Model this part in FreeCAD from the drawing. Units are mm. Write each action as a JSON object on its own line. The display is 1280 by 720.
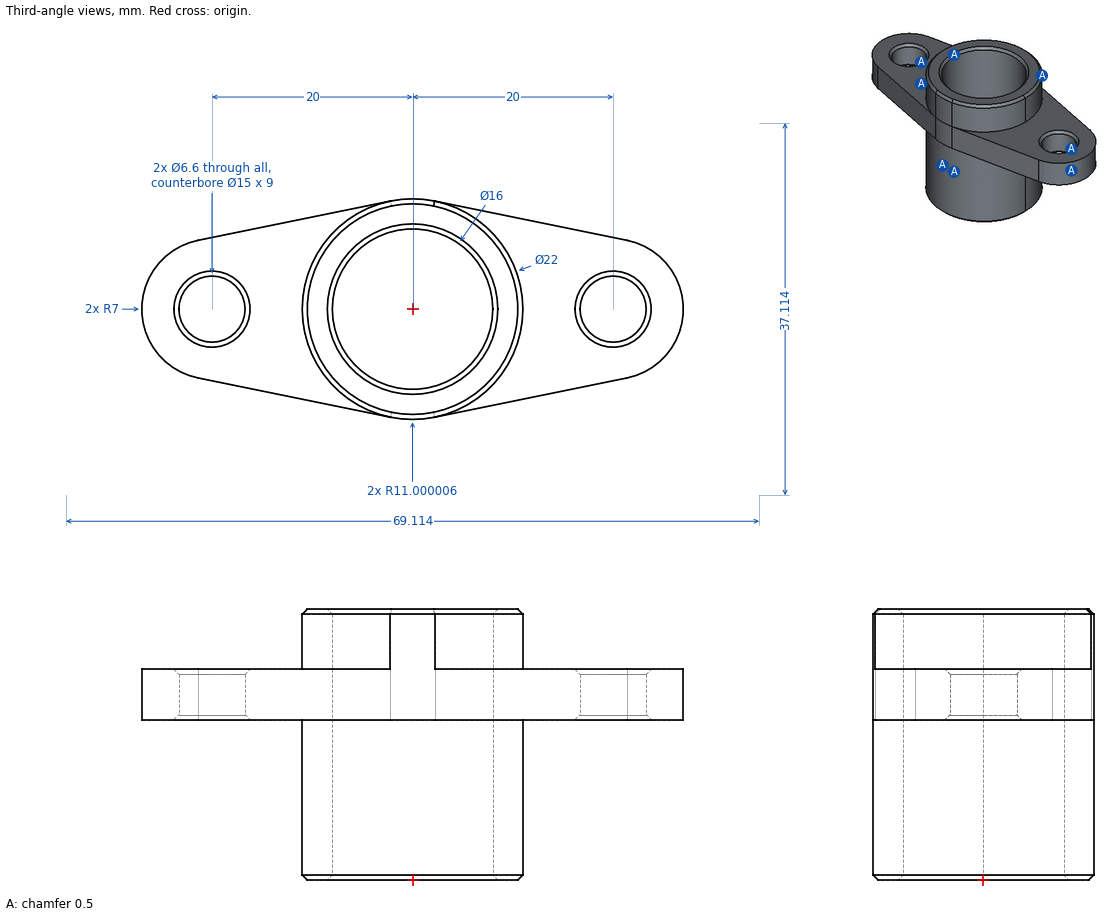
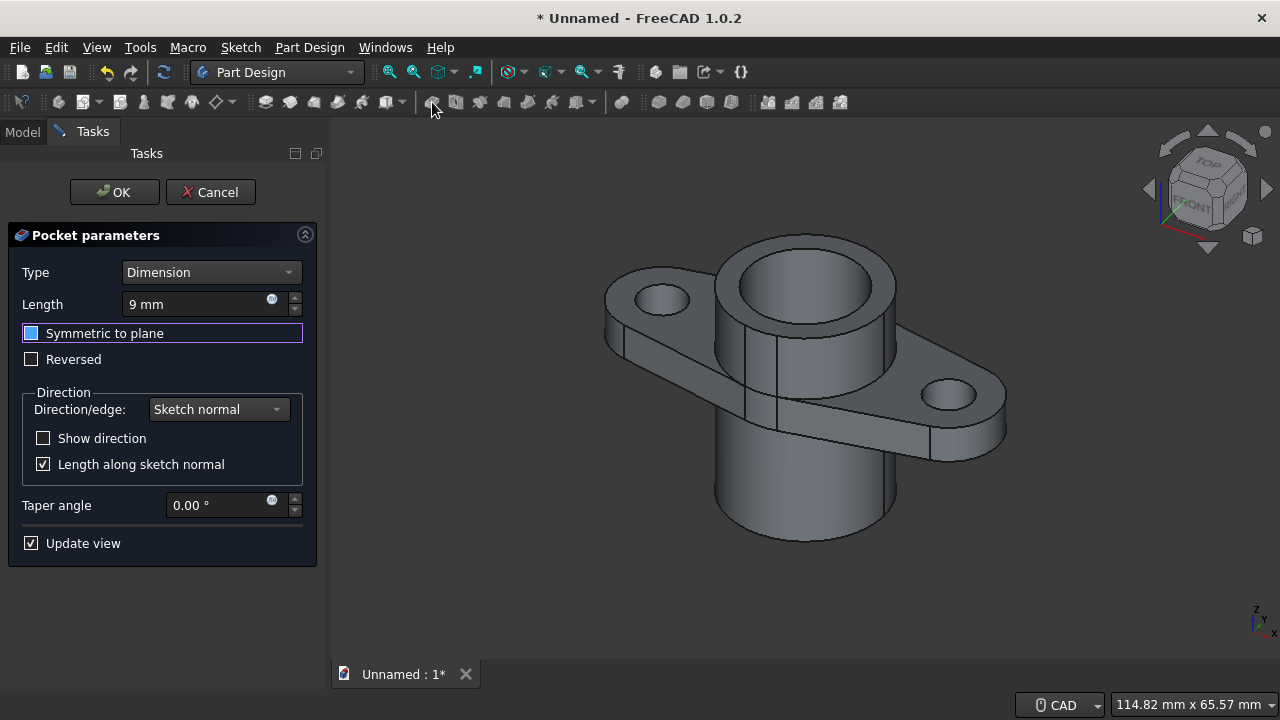
{"action": "left_click", "coordinate": [115, 192]}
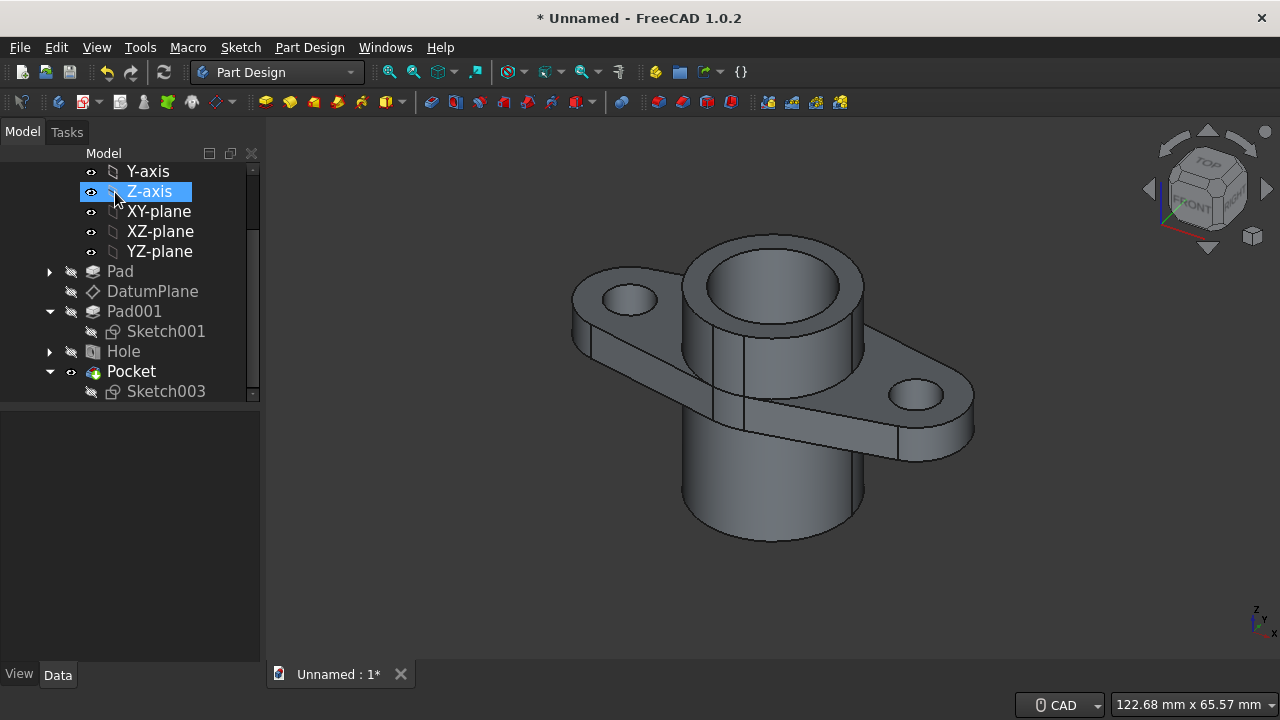
{"action": "scroll", "coordinate": [160, 287], "scroll_direction": "down", "scroll_amount": 3}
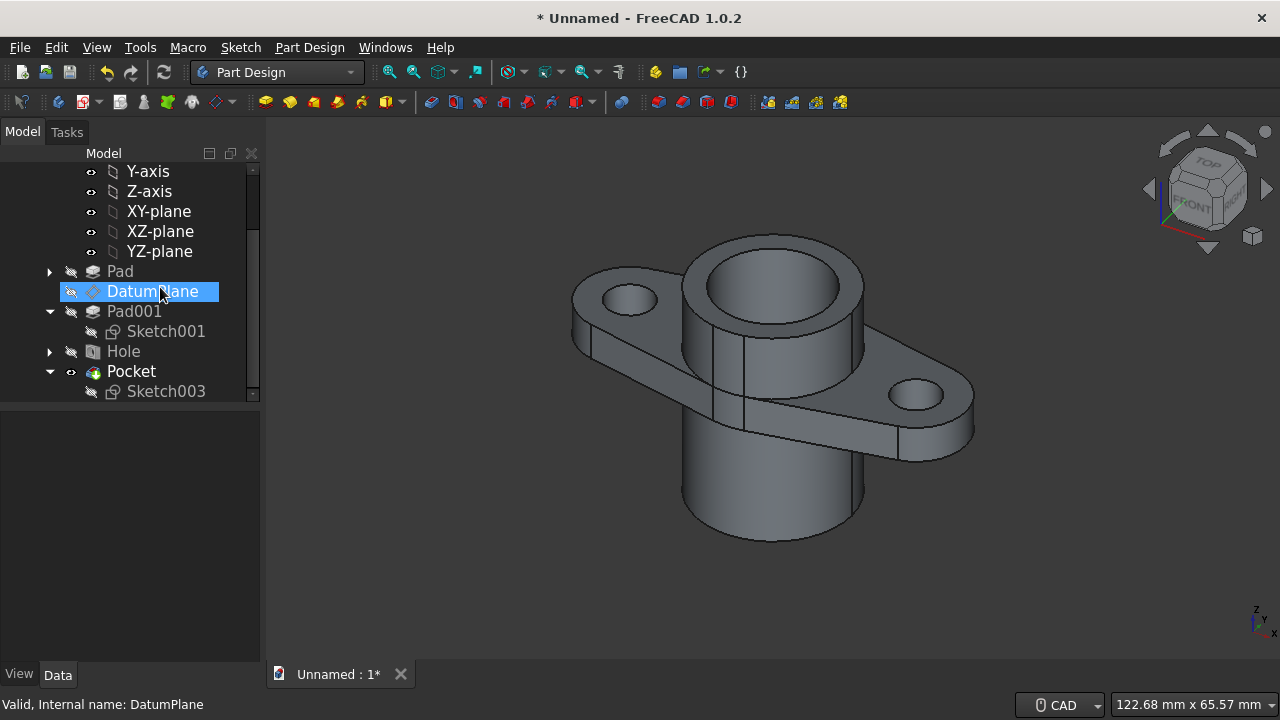
{"action": "scroll", "coordinate": [160, 287], "scroll_direction": "up", "scroll_amount": 15}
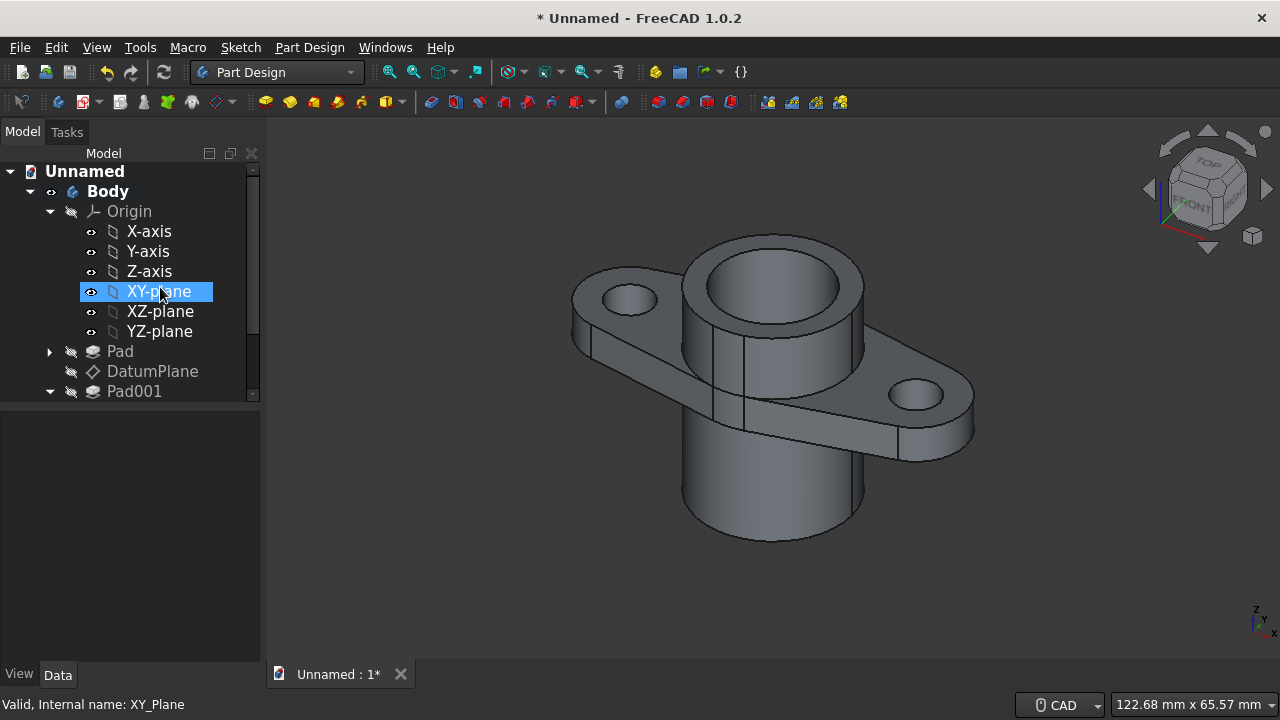
{"action": "left_click", "coordinate": [136, 292]}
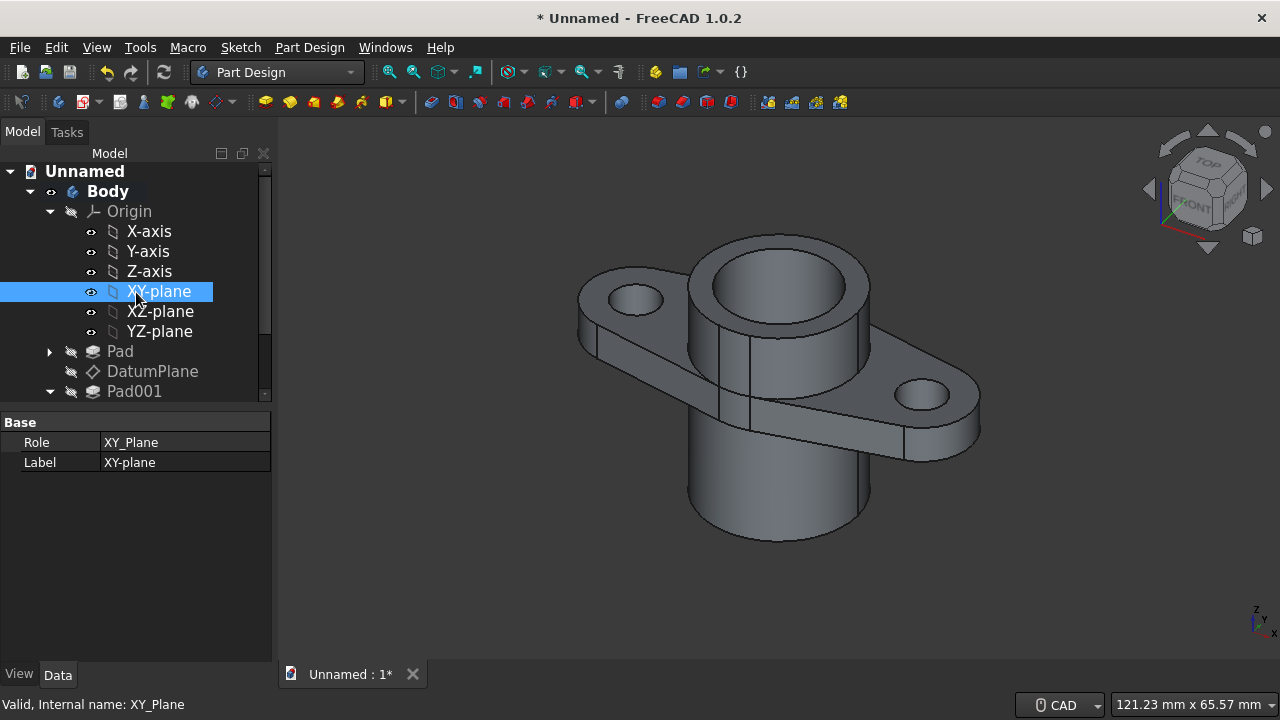
{"action": "left_click", "coordinate": [216, 102]}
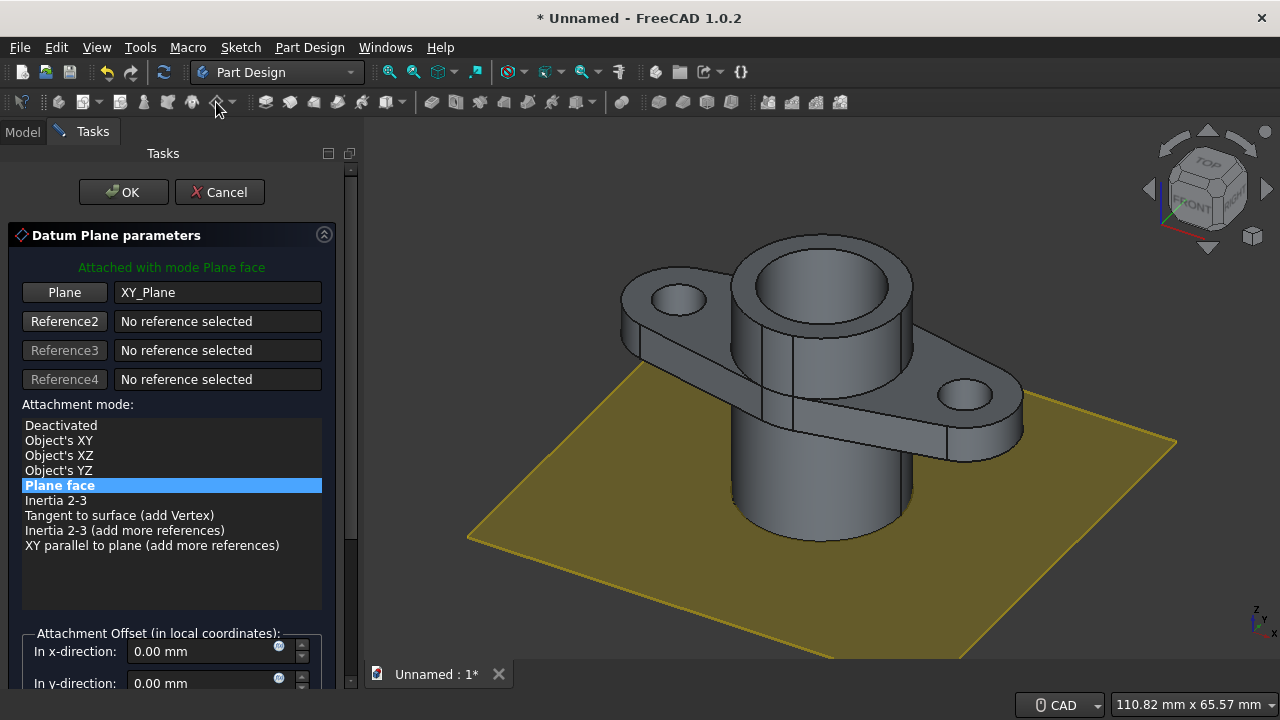
{"action": "scroll", "coordinate": [351, 426], "scroll_direction": "down", "scroll_amount": 2}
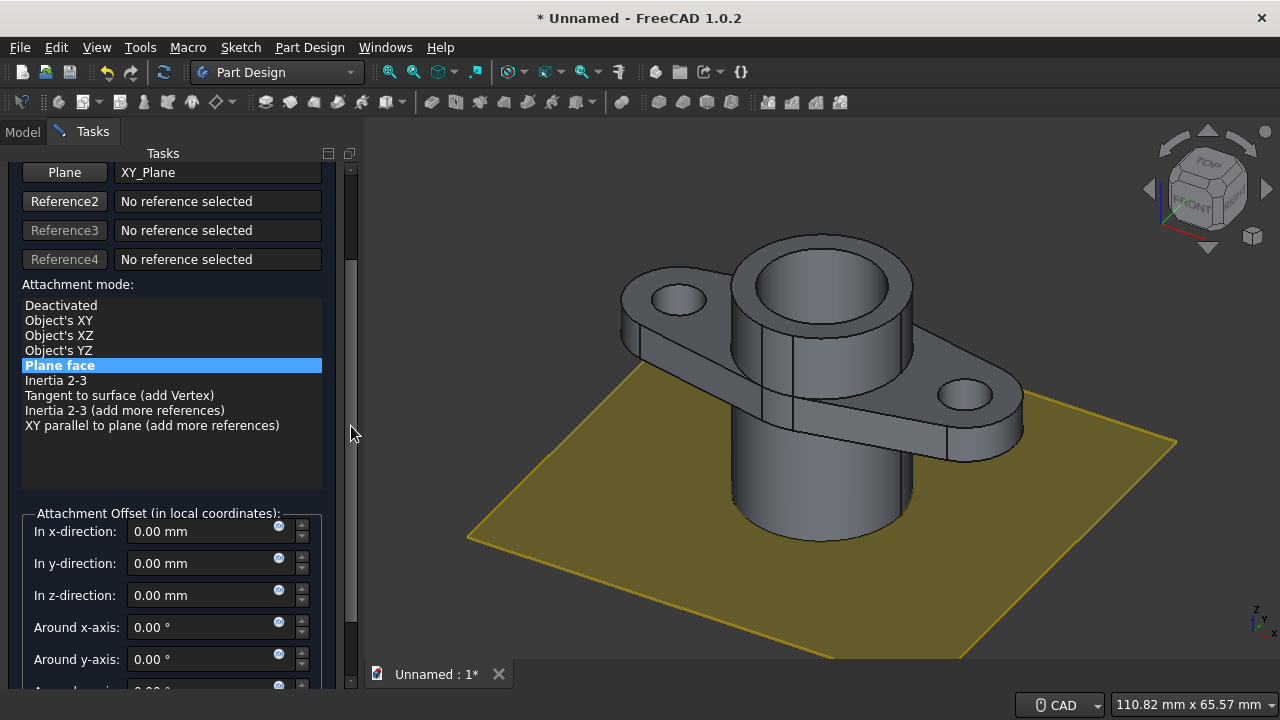
{"action": "triple_click", "coordinate": [210, 595]}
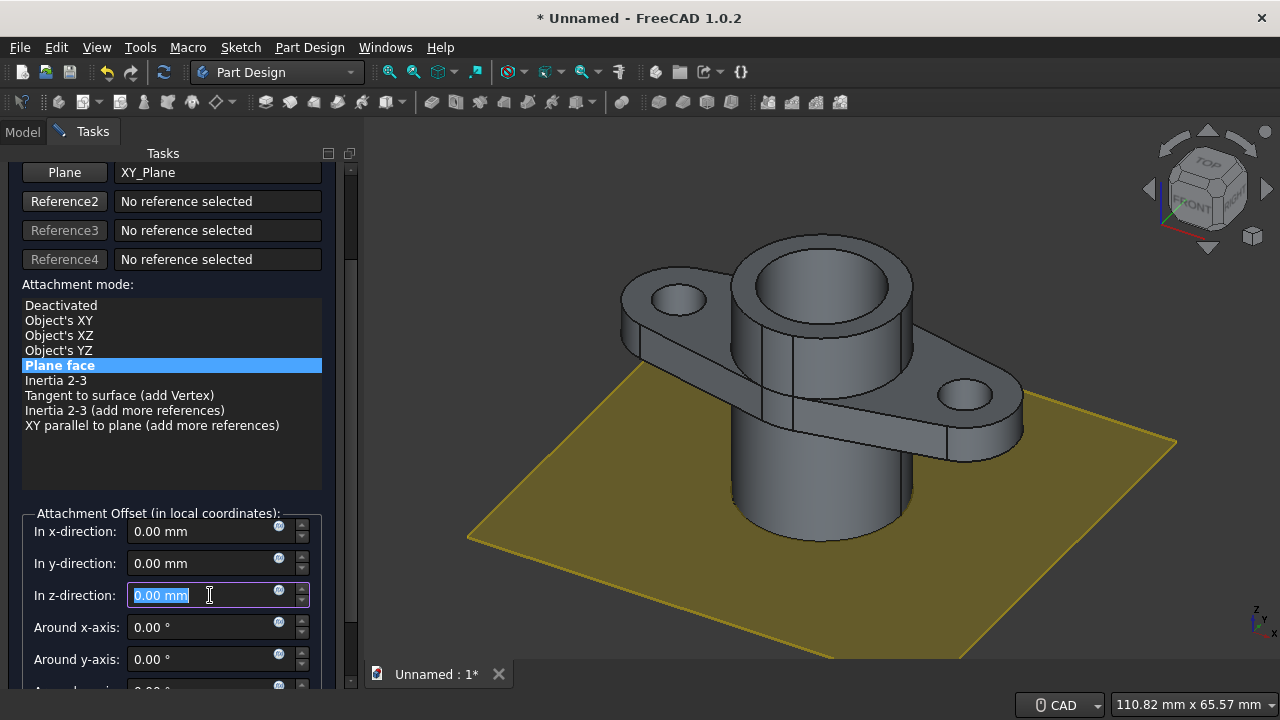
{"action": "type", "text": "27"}
{"action": "key", "text": "Tab"}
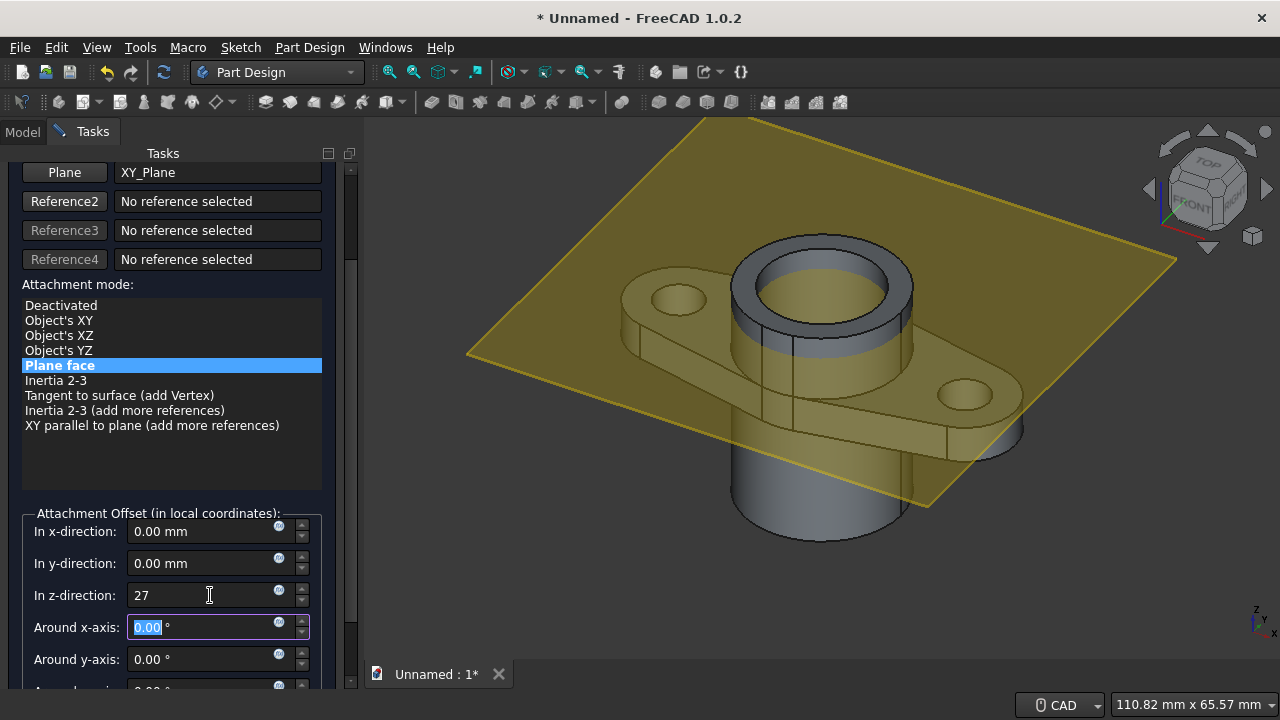
{"action": "scroll", "coordinate": [351, 426], "scroll_direction": "up", "scroll_amount": 3}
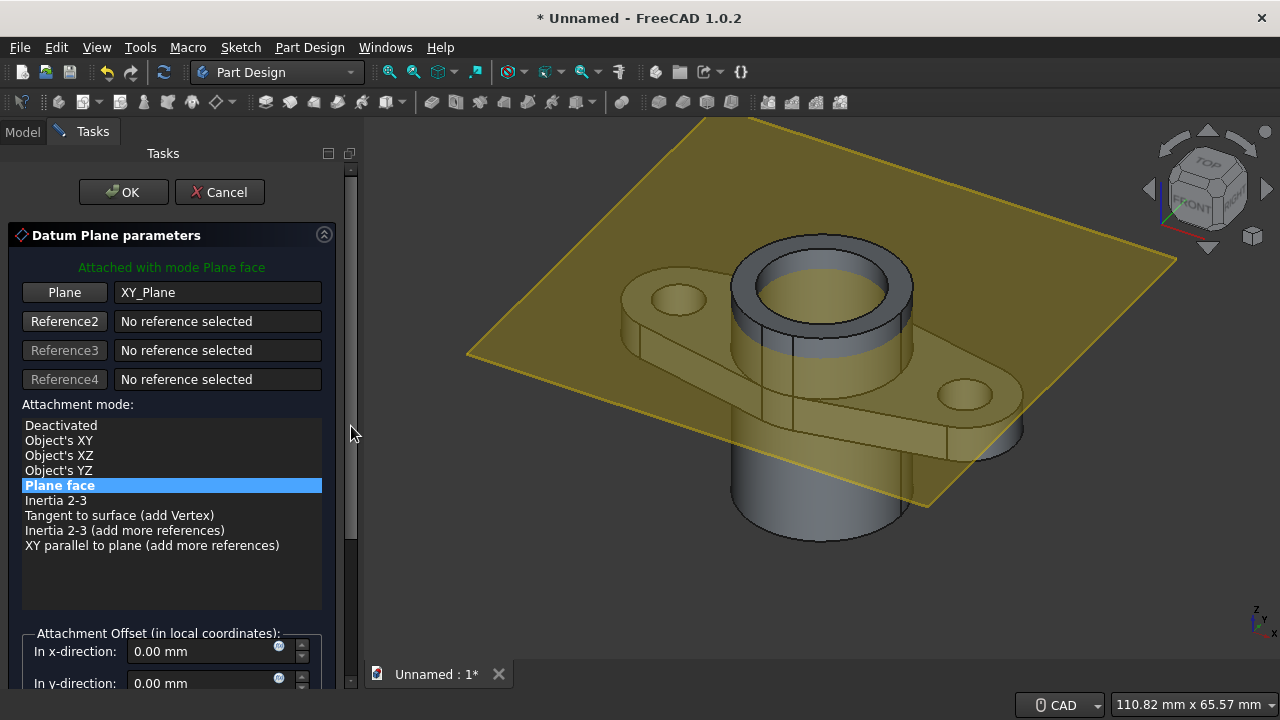
{"action": "left_click", "coordinate": [124, 192]}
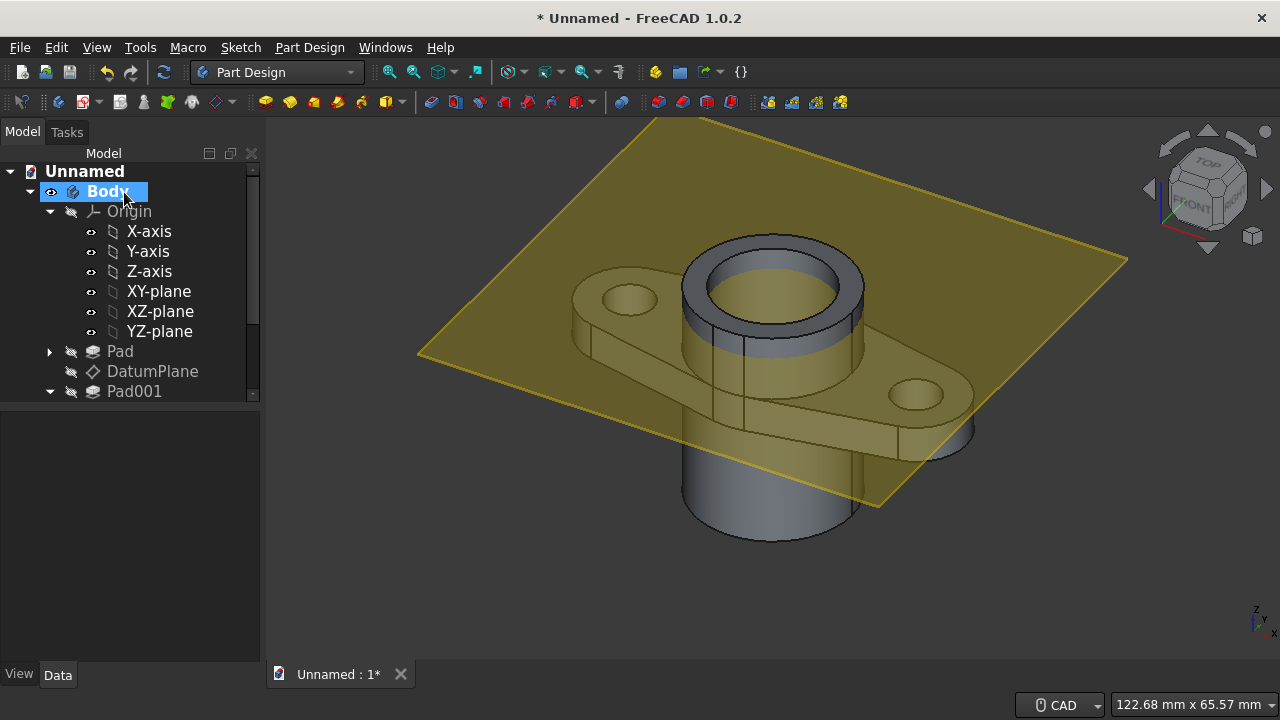
{"action": "scroll", "coordinate": [100, 287], "scroll_direction": "down", "scroll_amount": 3}